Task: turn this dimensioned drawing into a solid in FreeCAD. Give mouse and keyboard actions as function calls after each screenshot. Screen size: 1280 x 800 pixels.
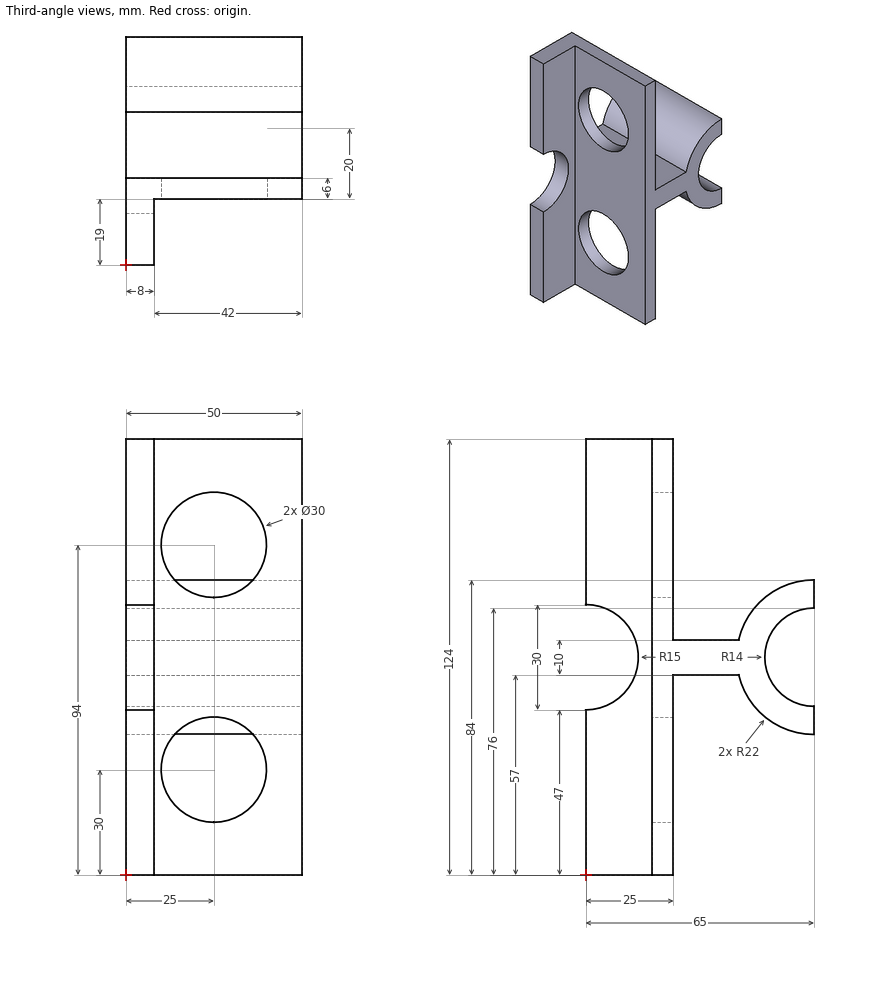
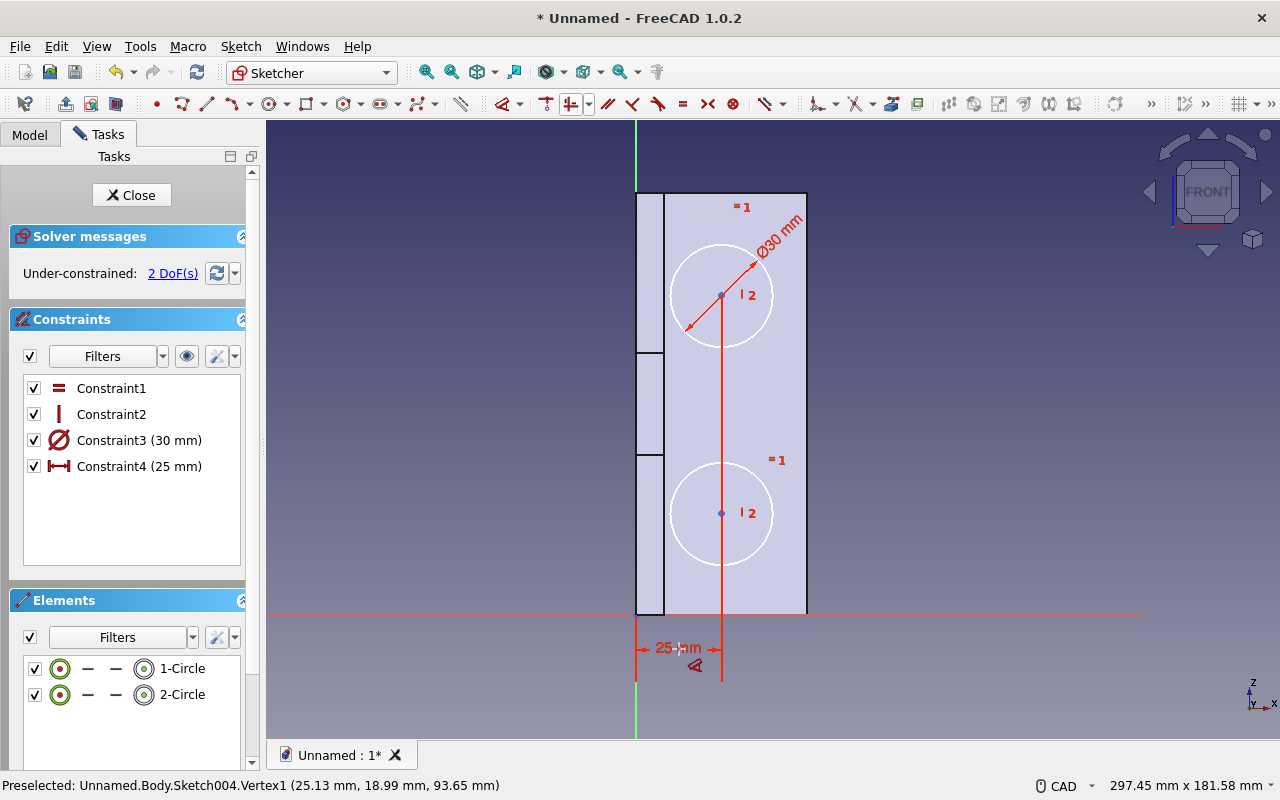
click(722, 296)
click(602, 456)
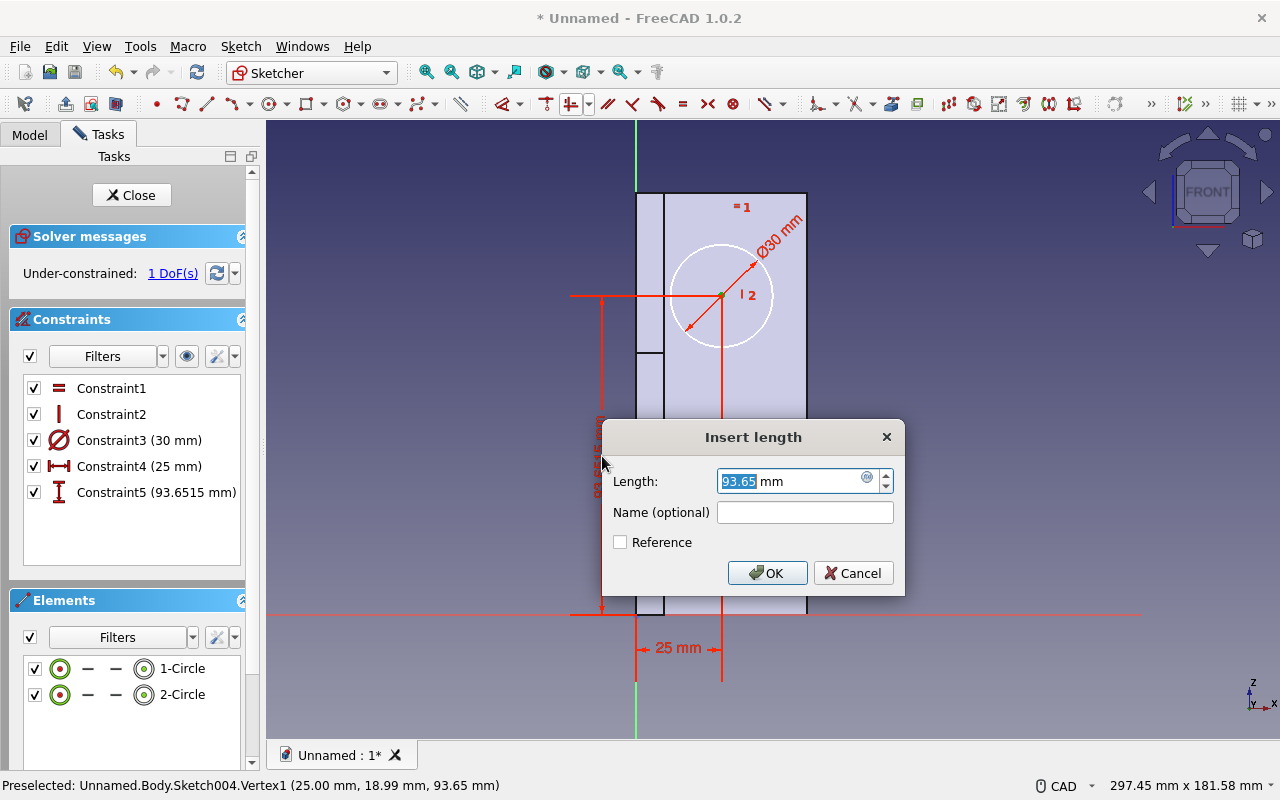
text(94)
key(Return)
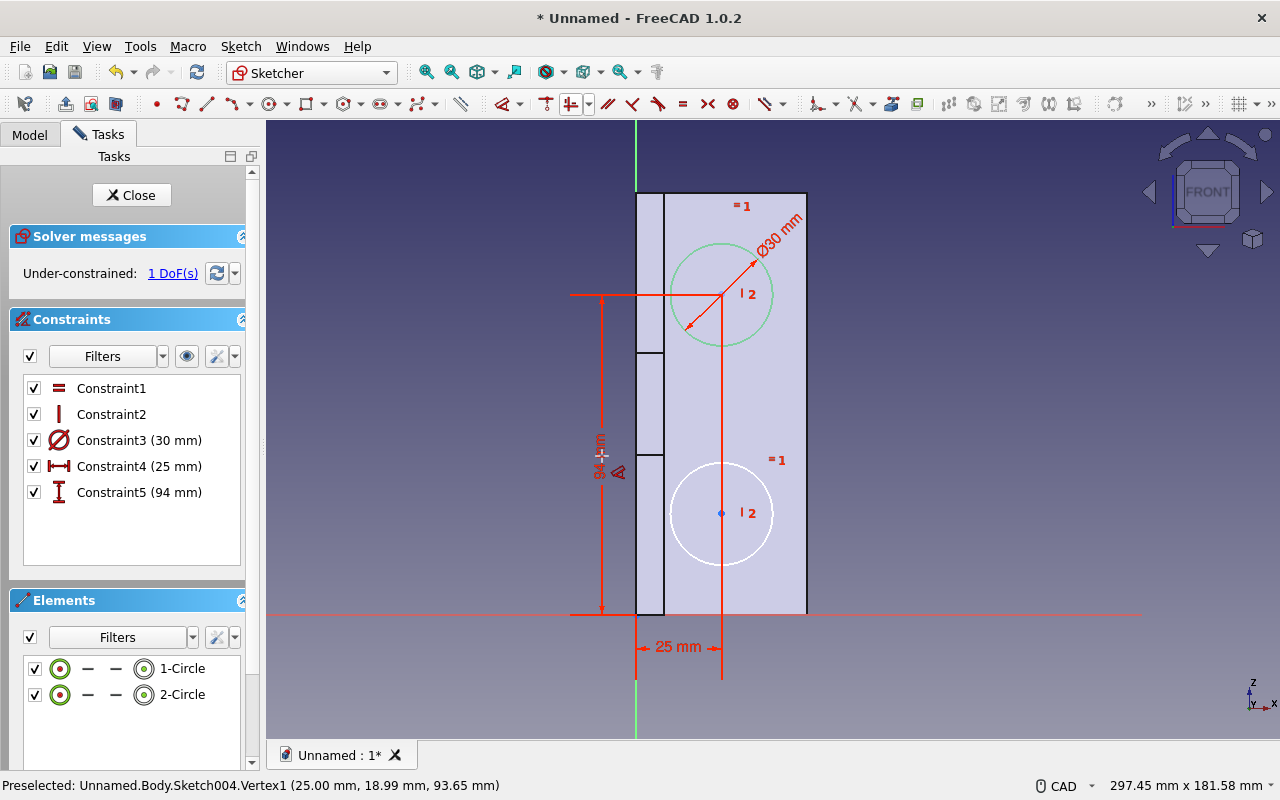
click(722, 514)
click(602, 565)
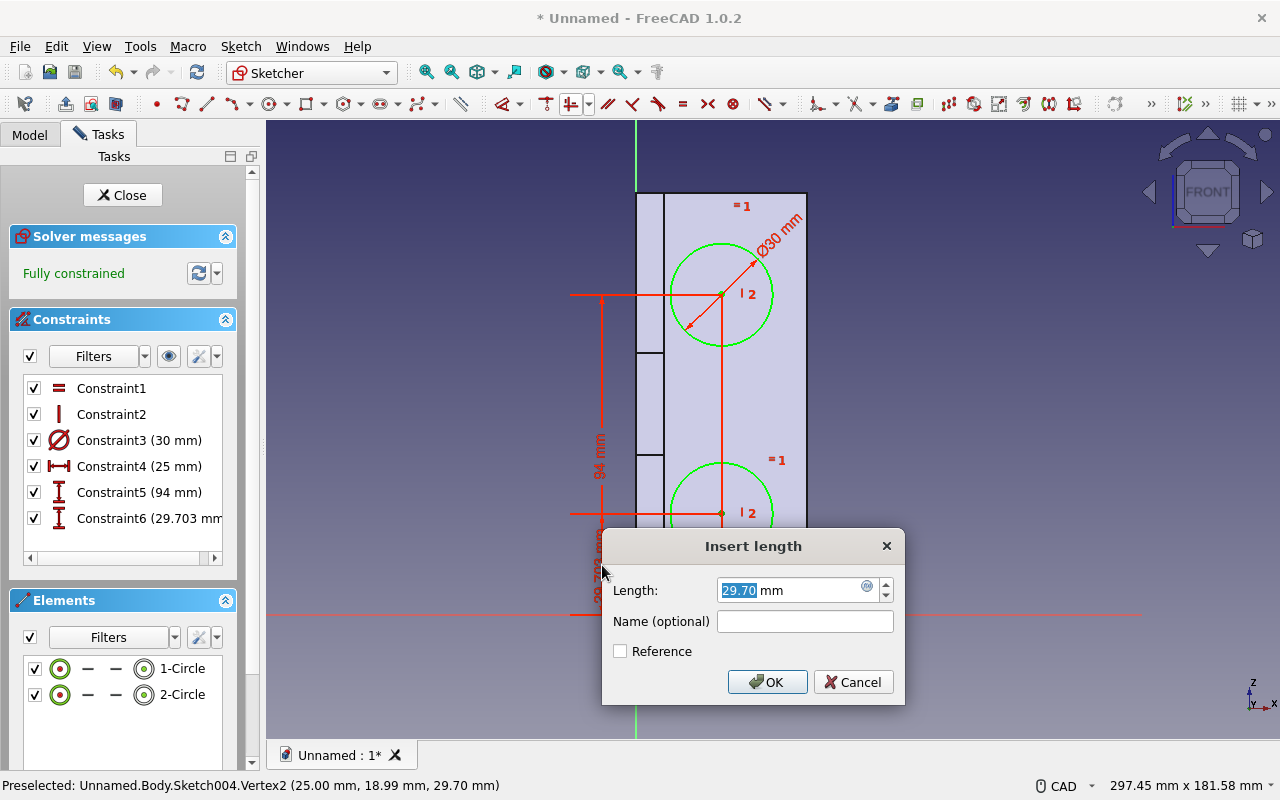
text(30)
key(Return)
key(Escape)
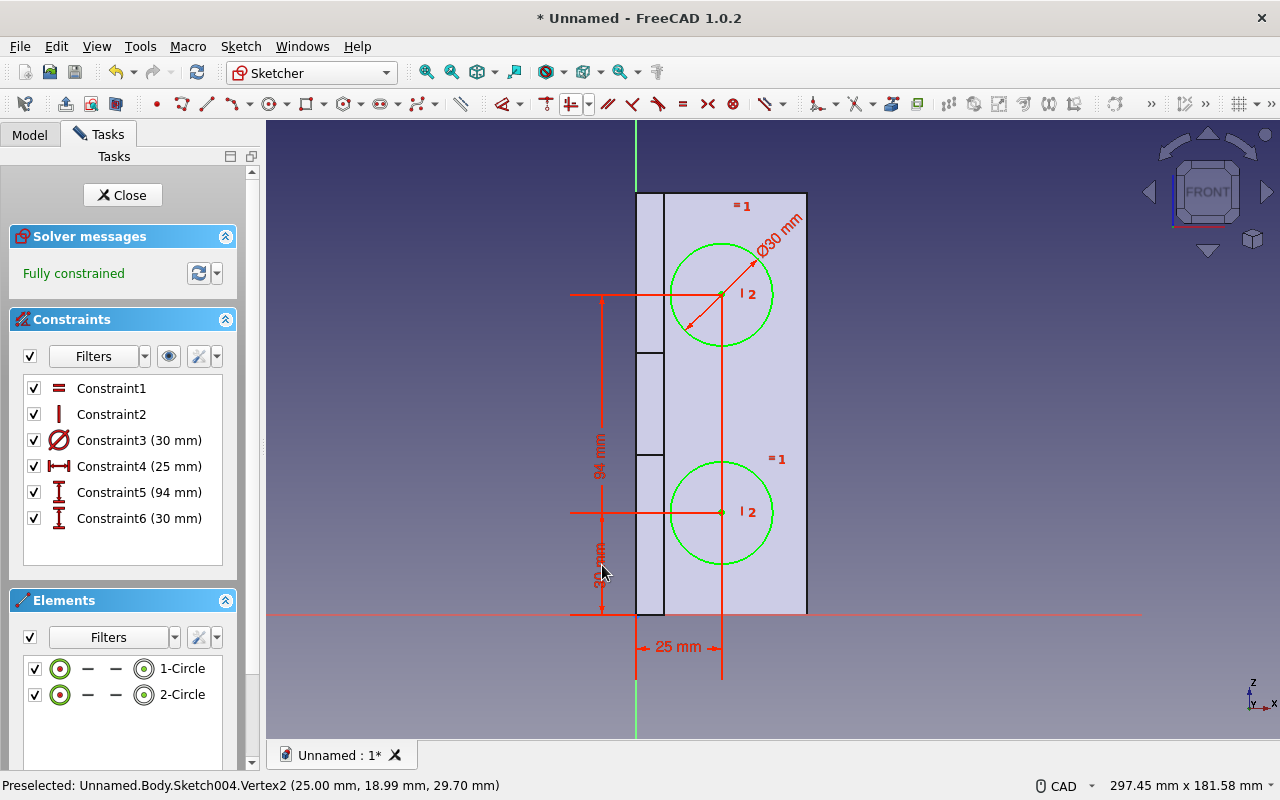
click(123, 195)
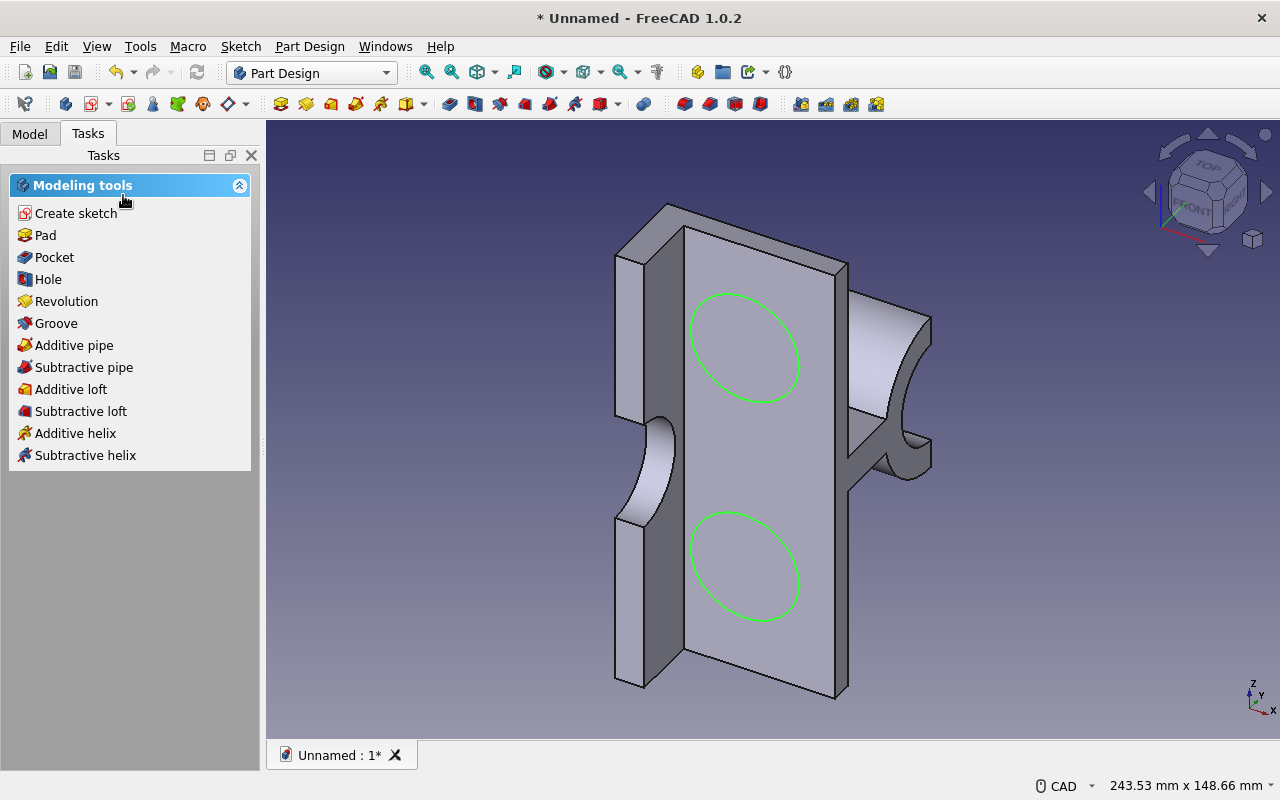
click(450, 104)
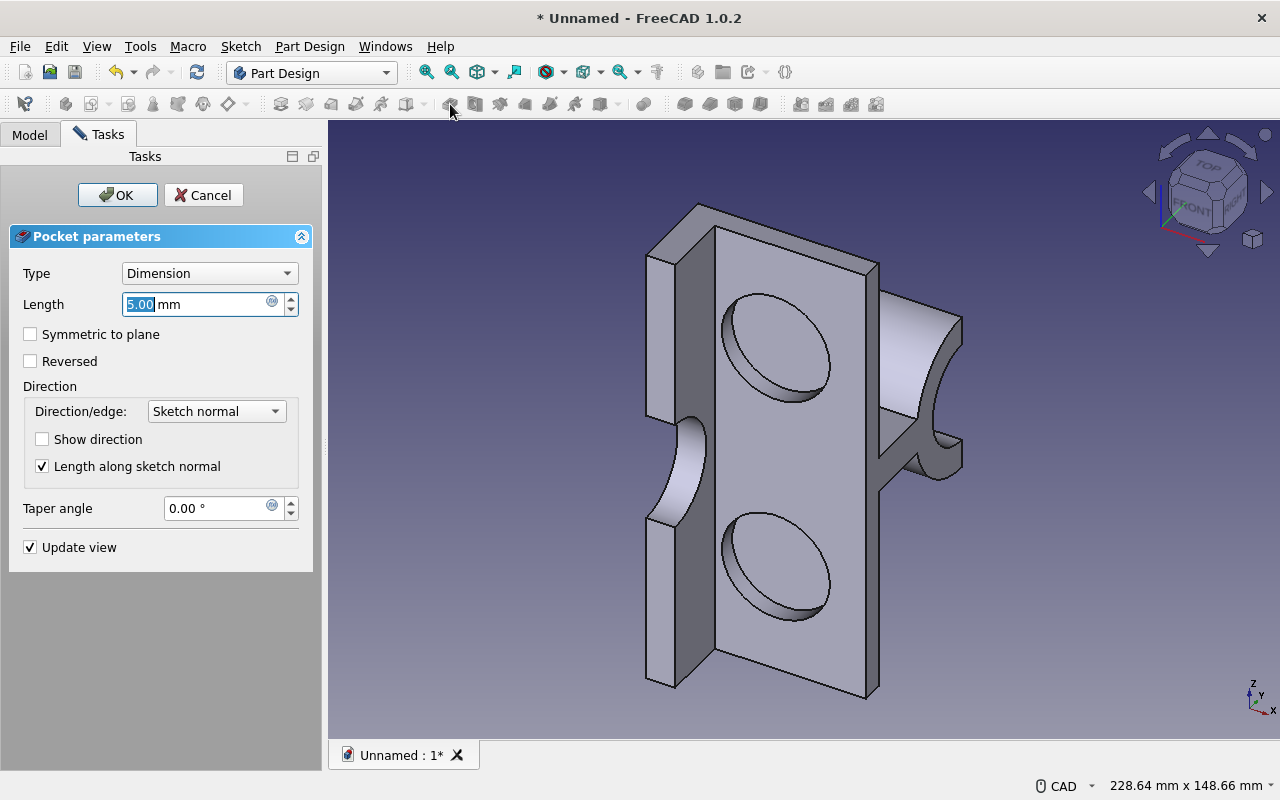
text(20)
key(Tab)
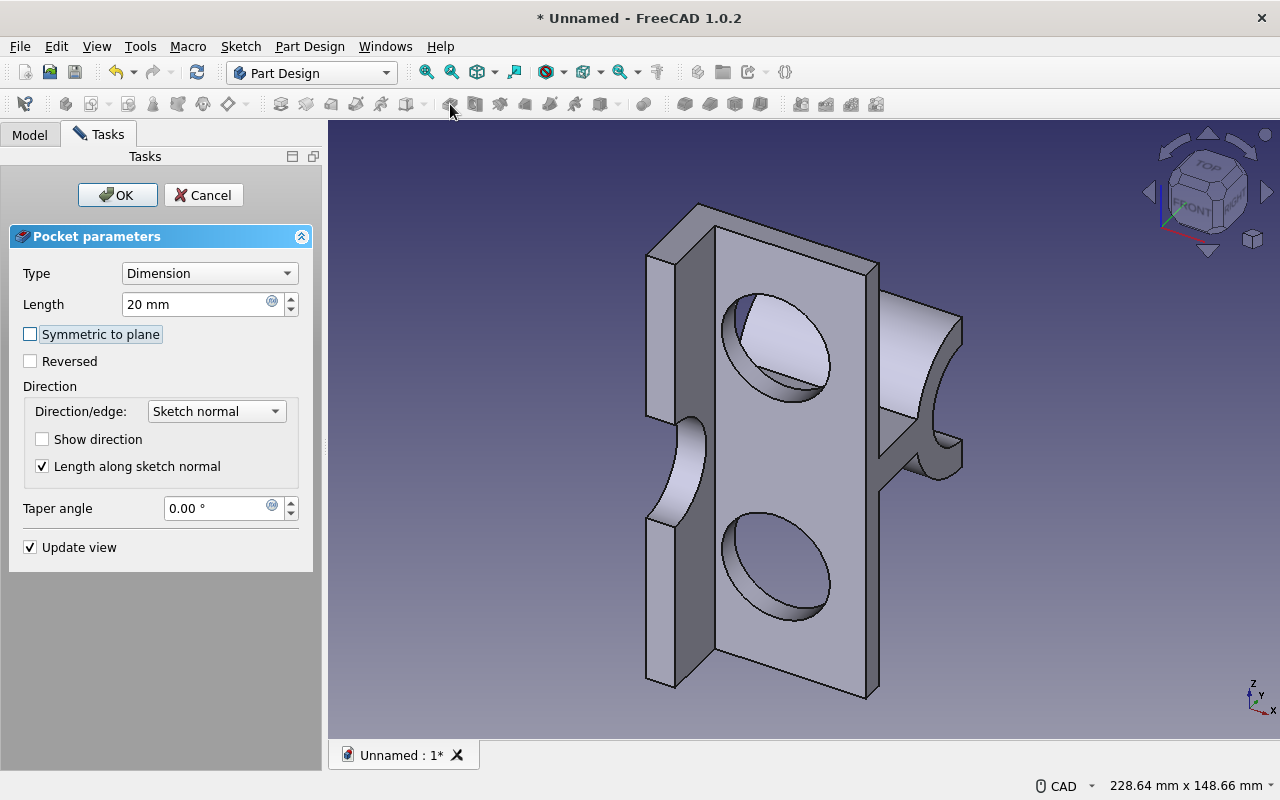
click(118, 195)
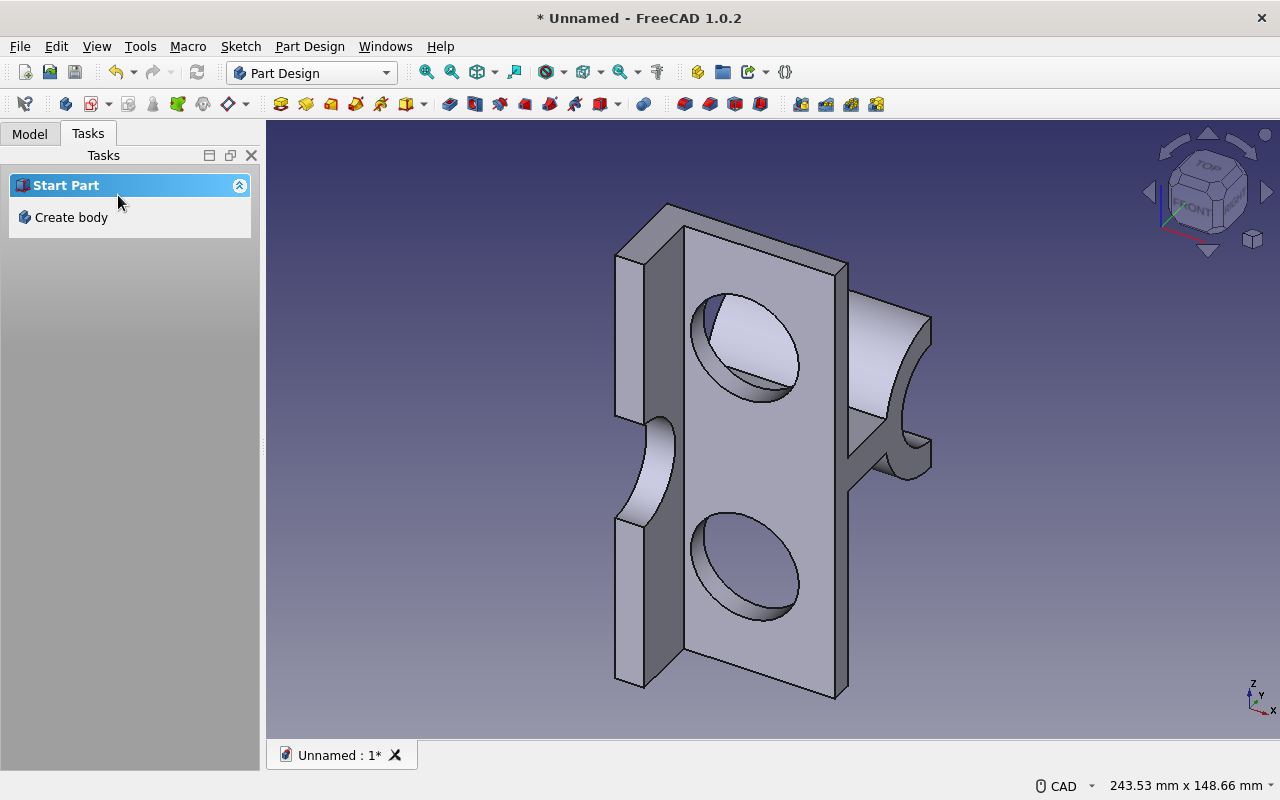
key(0)